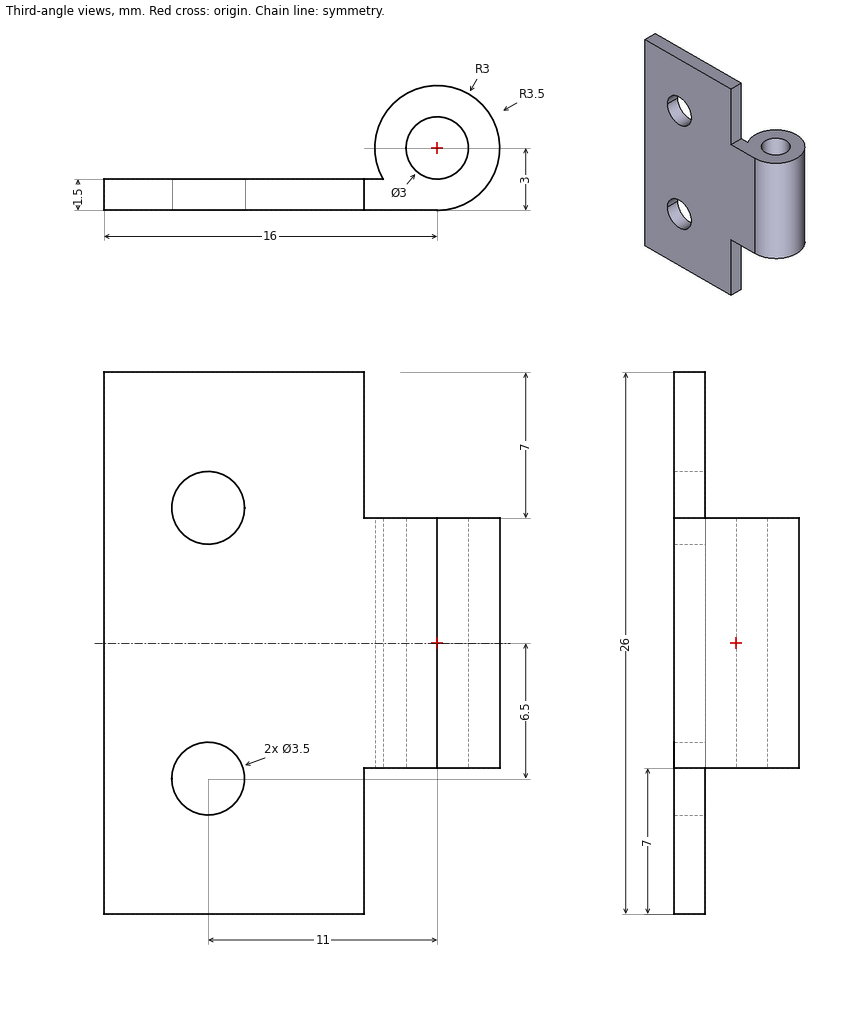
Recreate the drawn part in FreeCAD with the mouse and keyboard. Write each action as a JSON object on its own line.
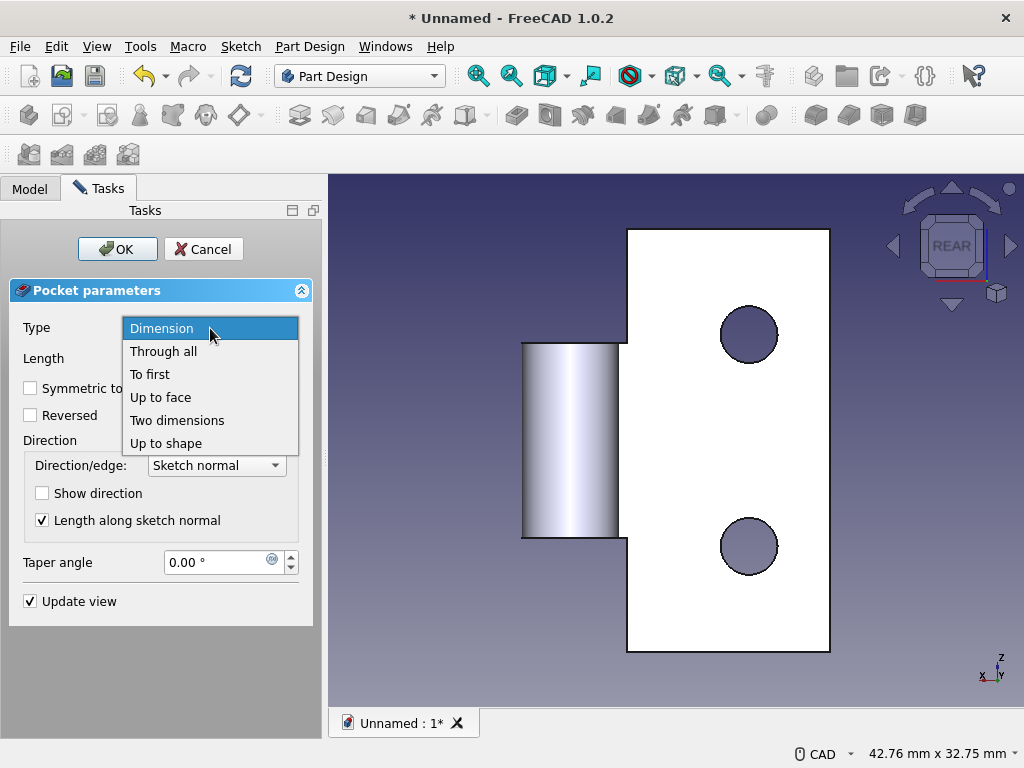
{"action": "left_click", "coordinate": [208, 352]}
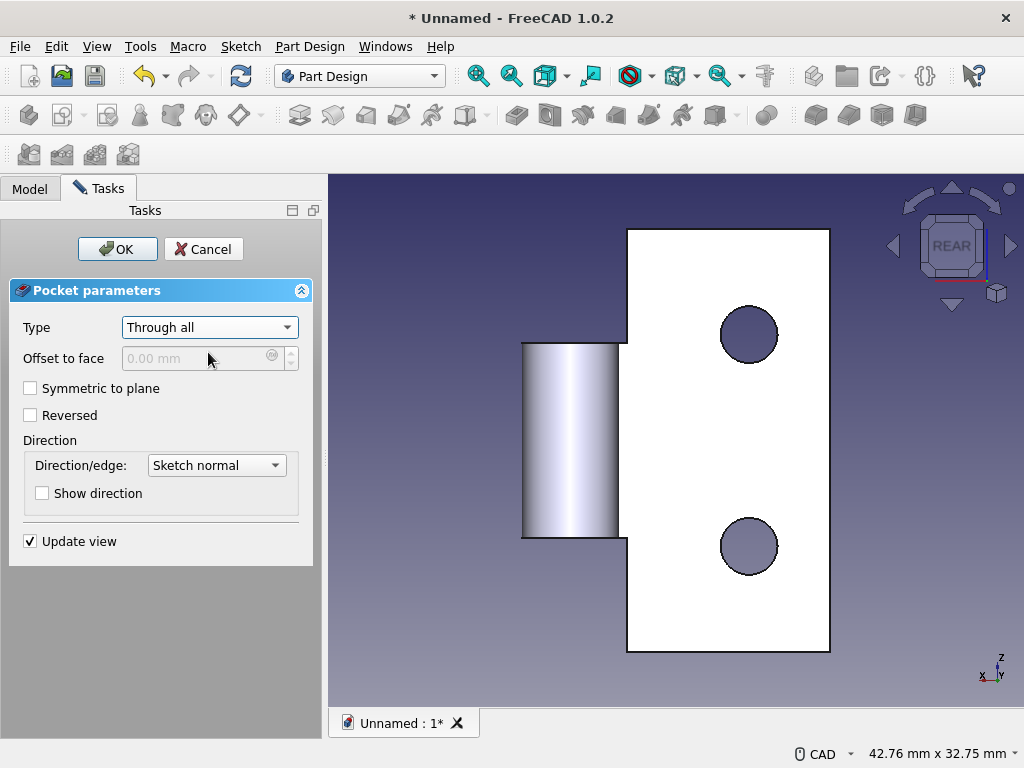
{"action": "left_click", "coordinate": [118, 249]}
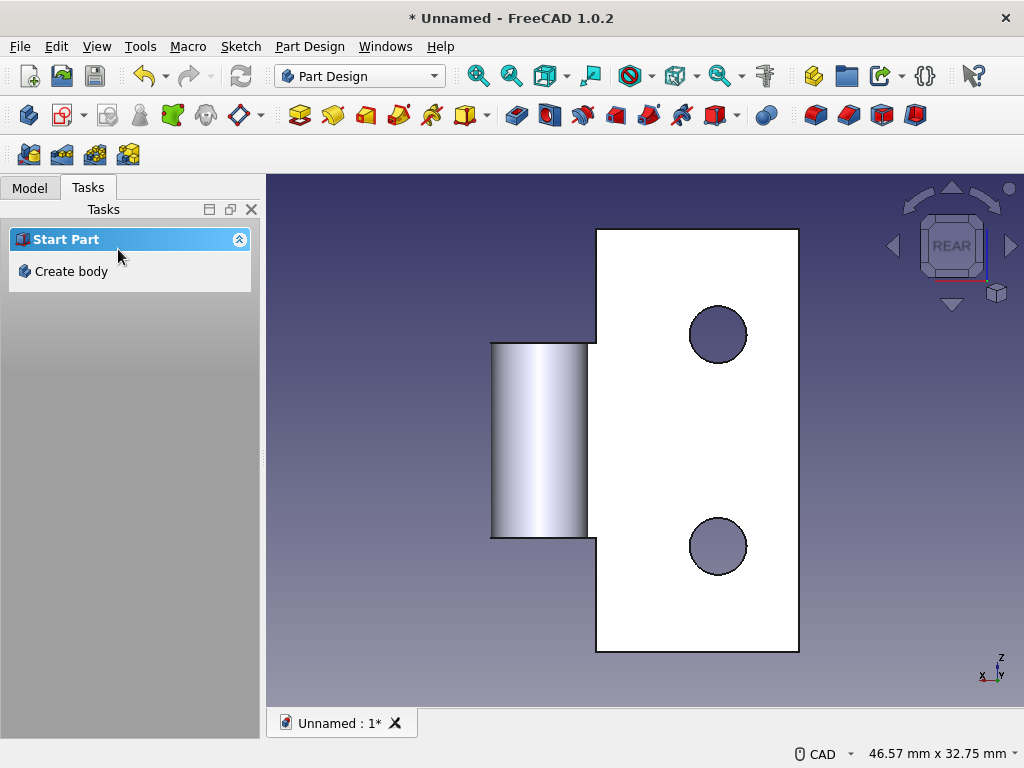
{"action": "key", "text": "0"}